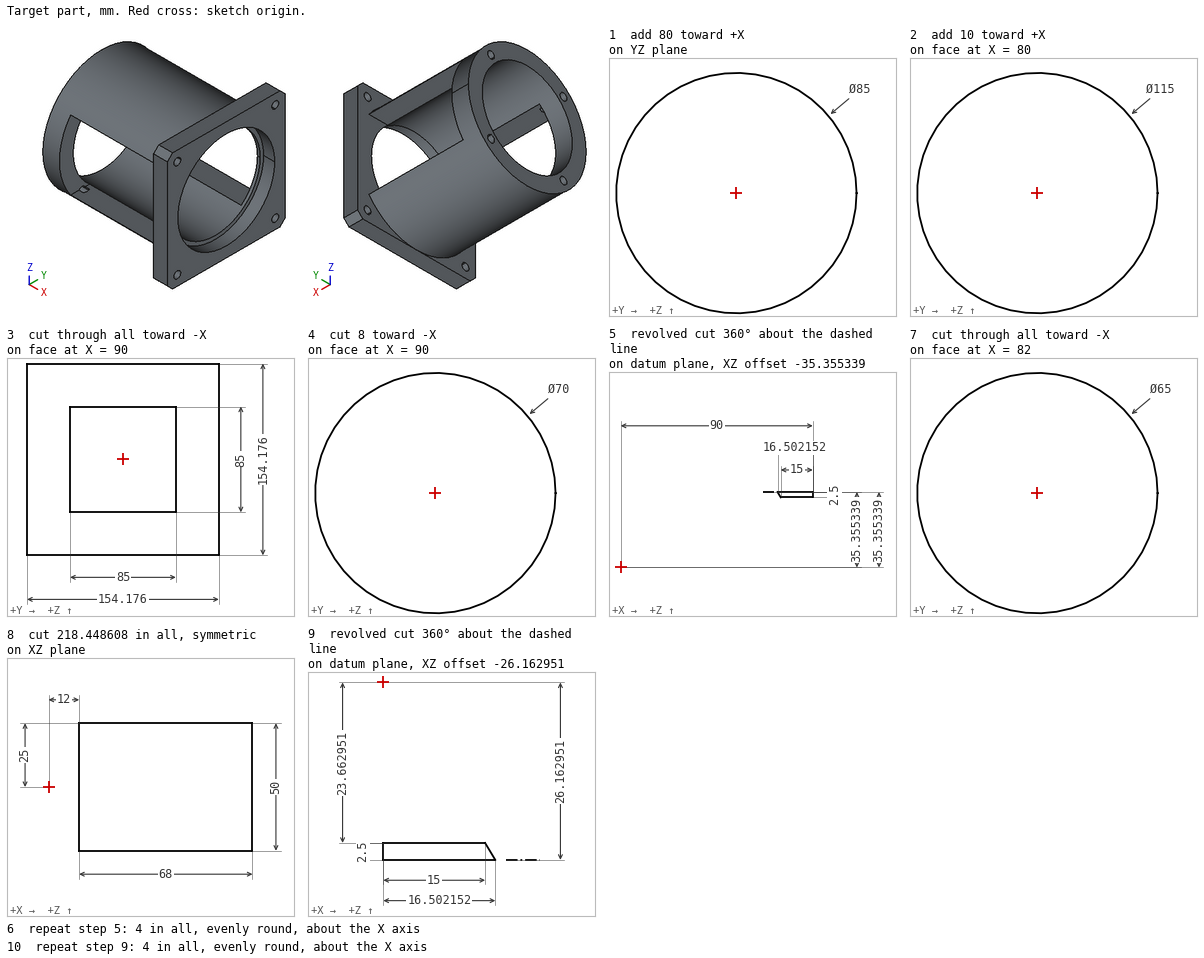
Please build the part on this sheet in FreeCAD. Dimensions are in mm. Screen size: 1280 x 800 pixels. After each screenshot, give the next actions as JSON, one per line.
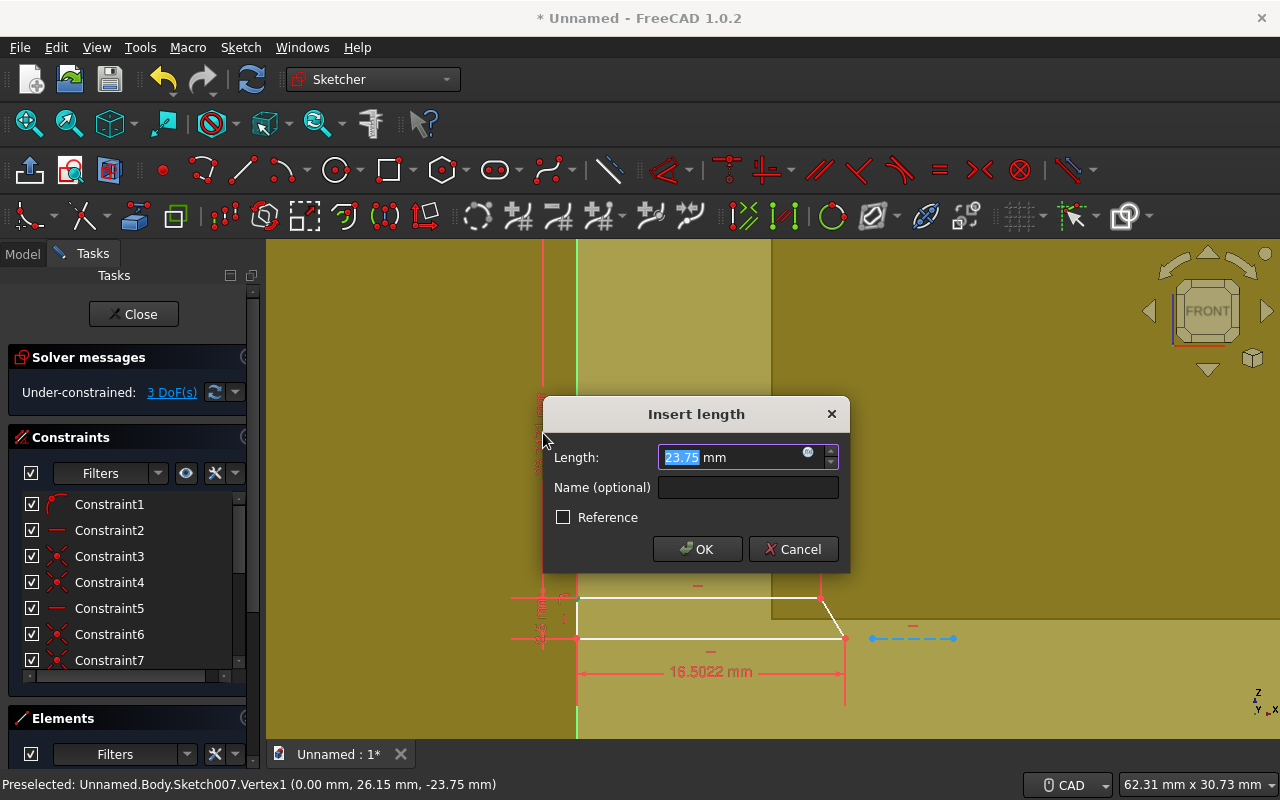
{"action": "type", "text": "23.662951"}
{"action": "key", "text": "Return"}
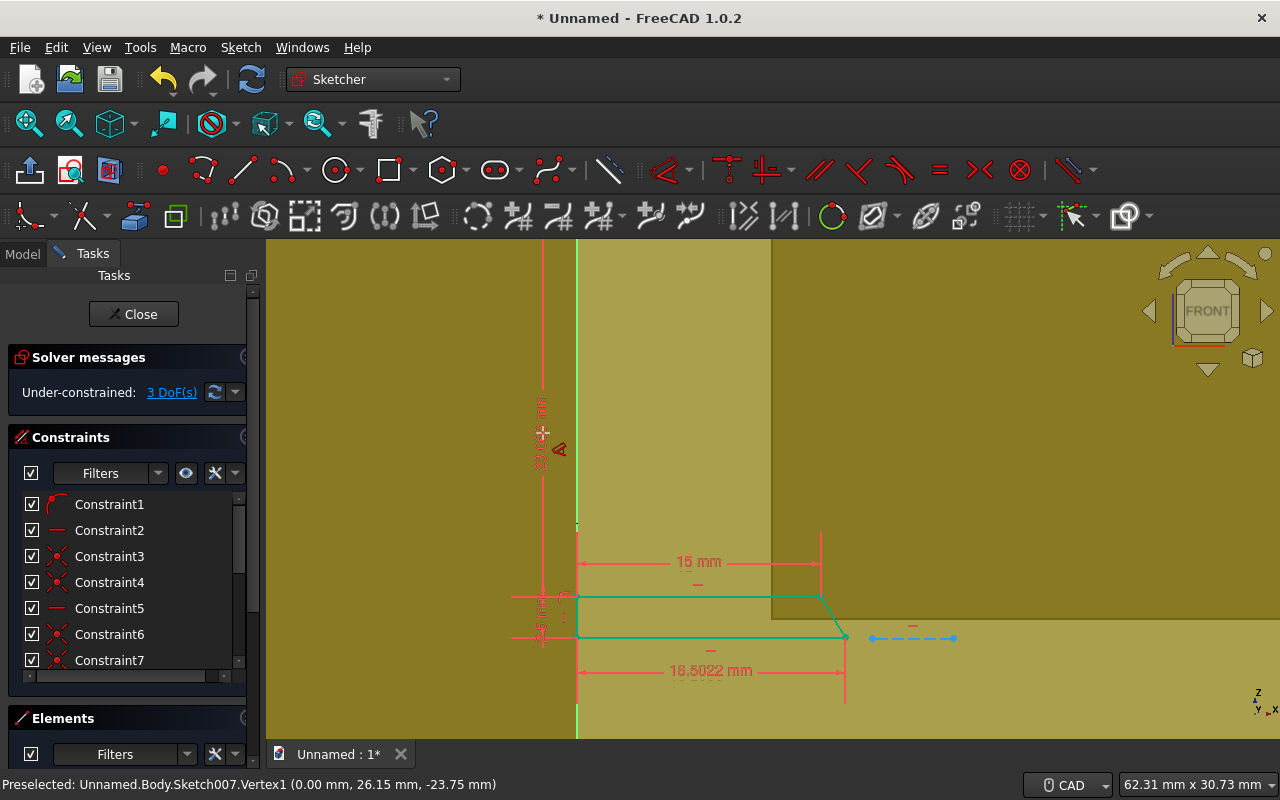
{"action": "left_click", "coordinate": [873, 638]}
{"action": "left_click", "coordinate": [543, 453]}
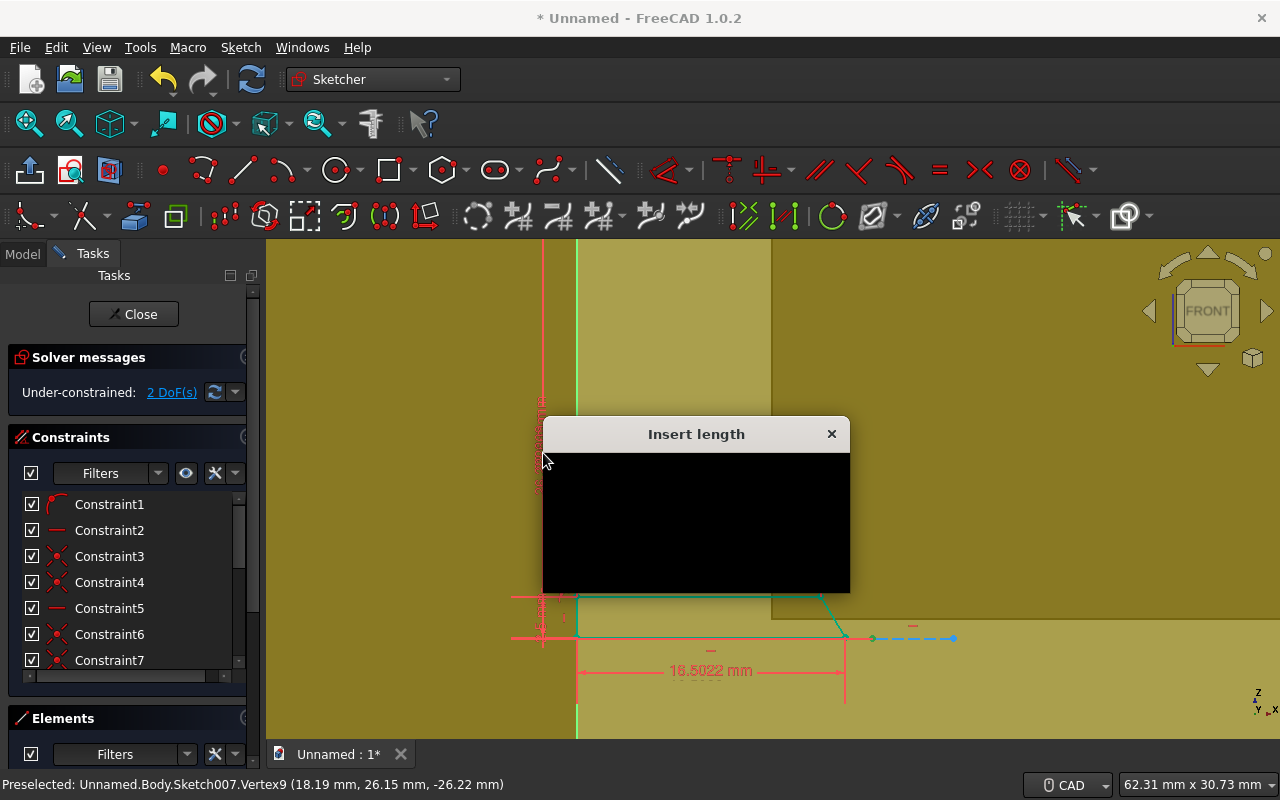
{"action": "type", "text": "26.162951"}
{"action": "key", "text": "Return"}
{"action": "key", "text": "Escape"}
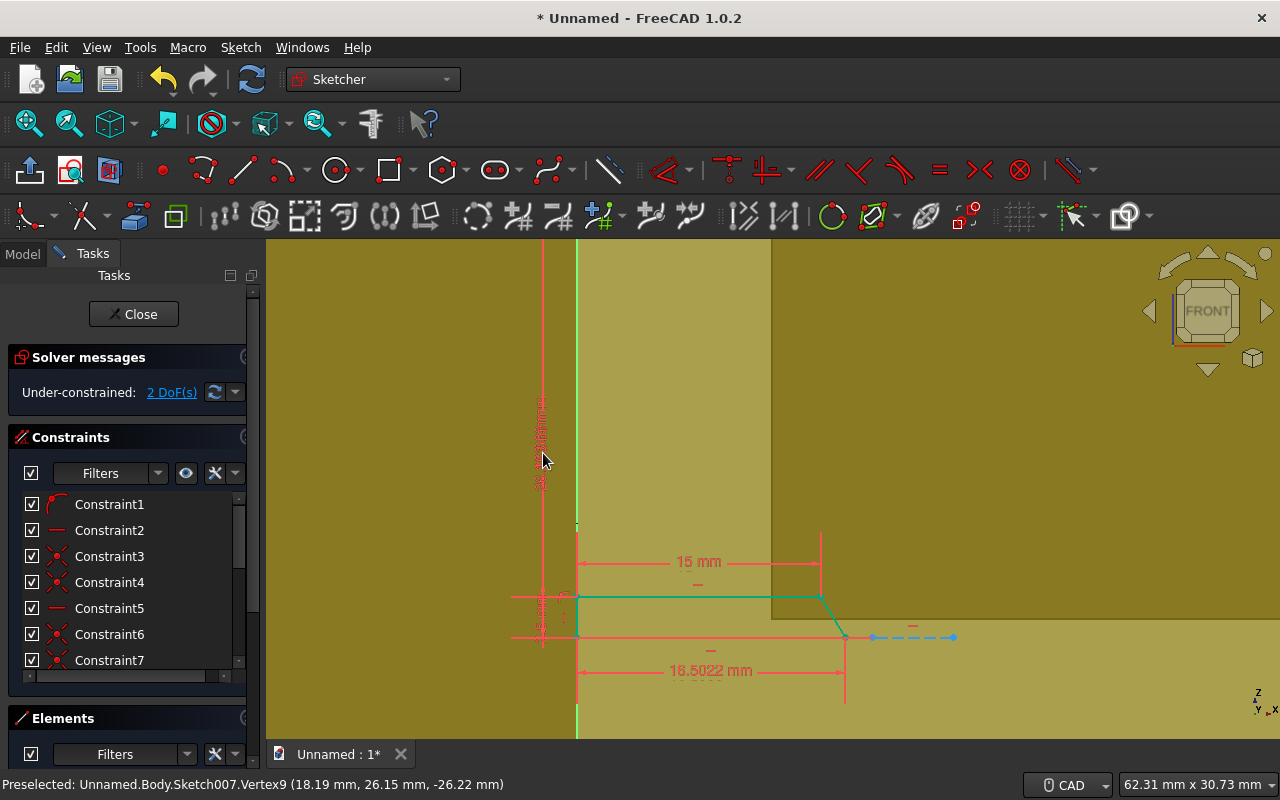
{"action": "left_click", "coordinate": [134, 314]}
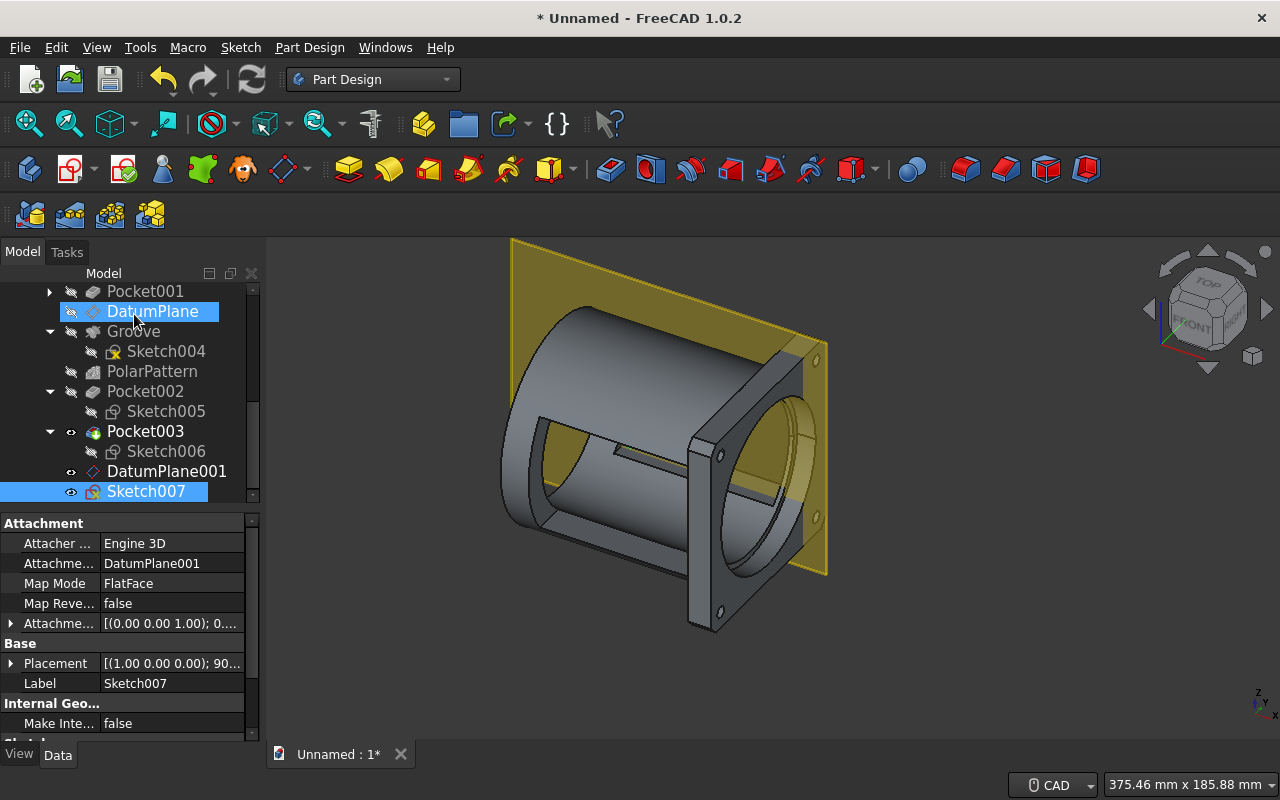
{"action": "left_click", "coordinate": [692, 170]}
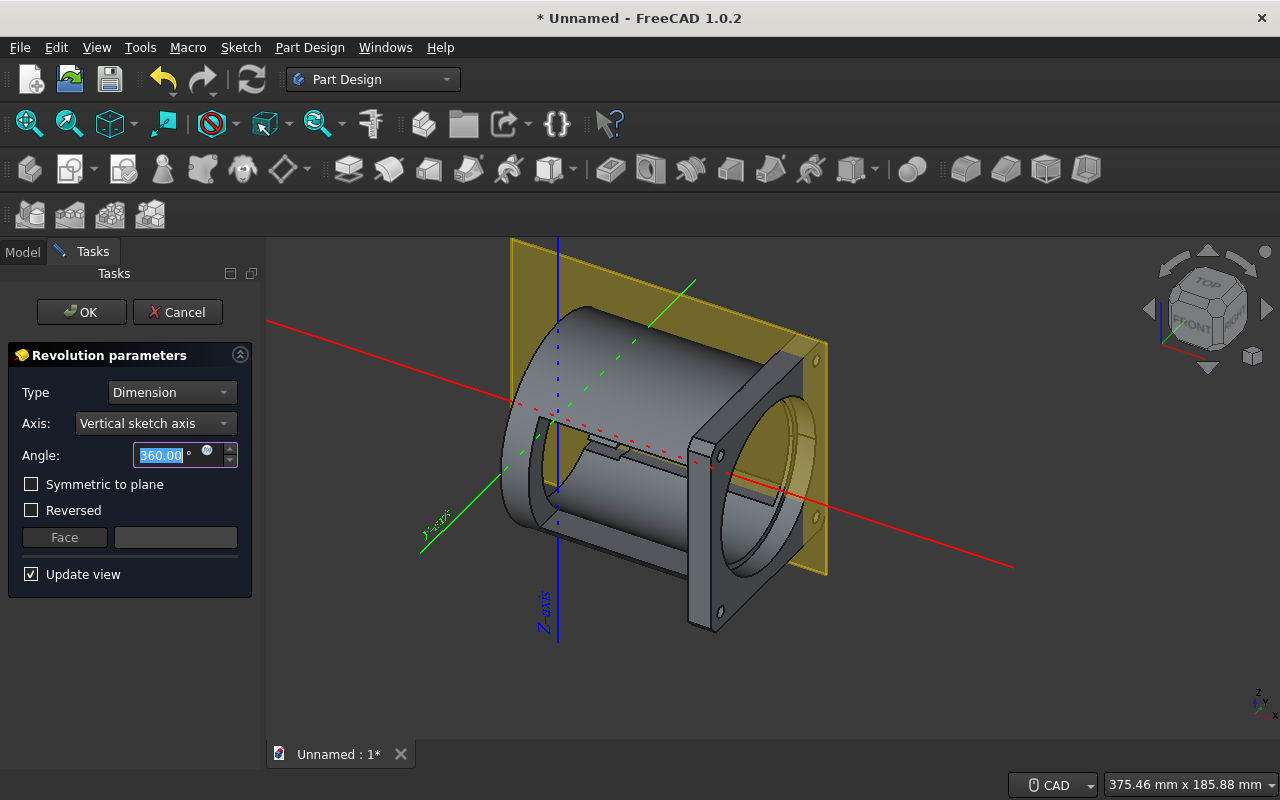
{"action": "left_click", "coordinate": [156, 424]}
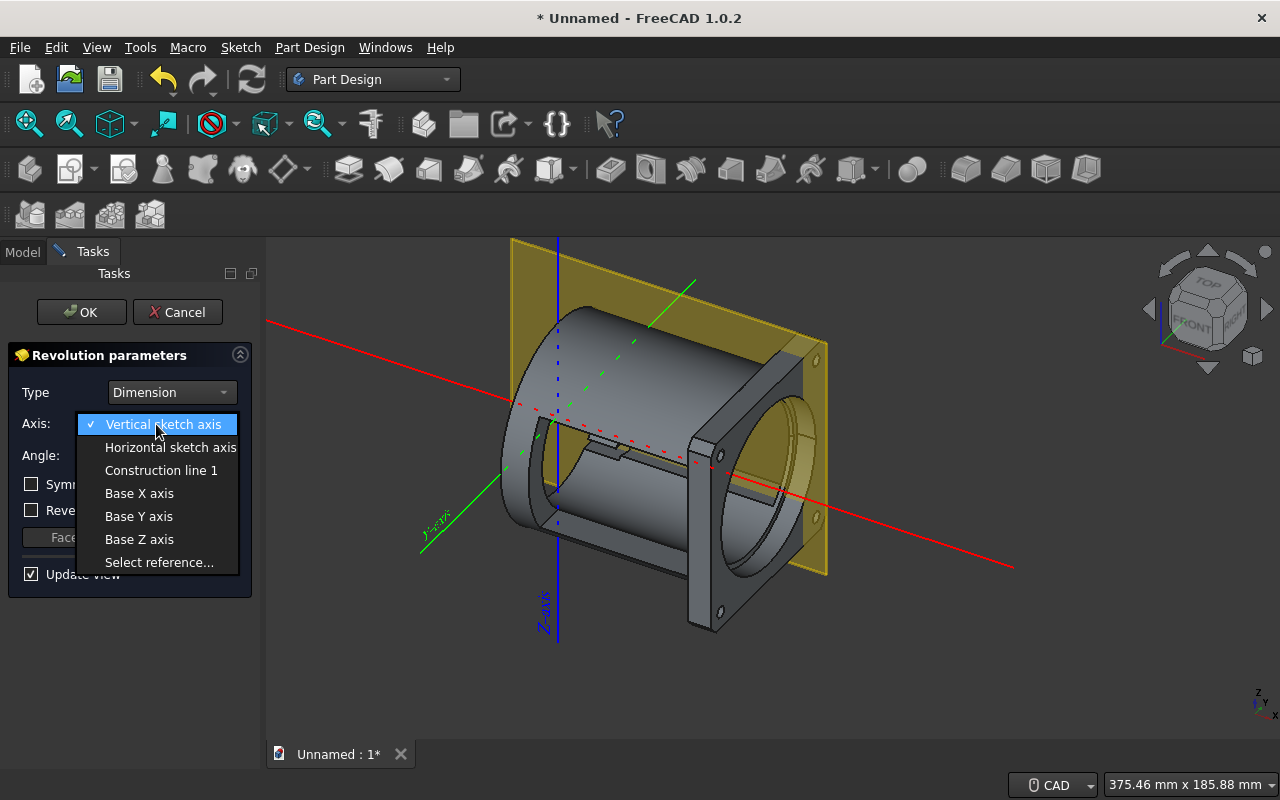
{"action": "left_click", "coordinate": [156, 470]}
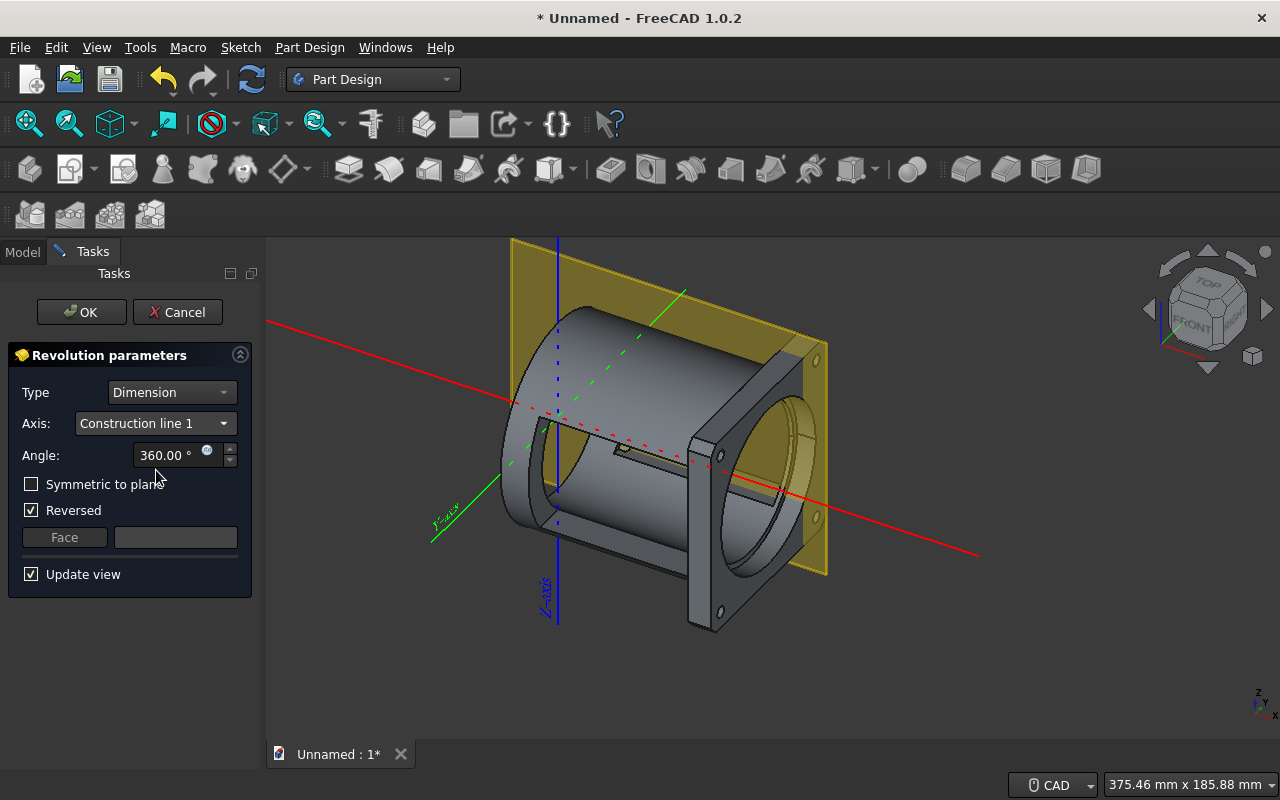
{"action": "left_click", "coordinate": [82, 312]}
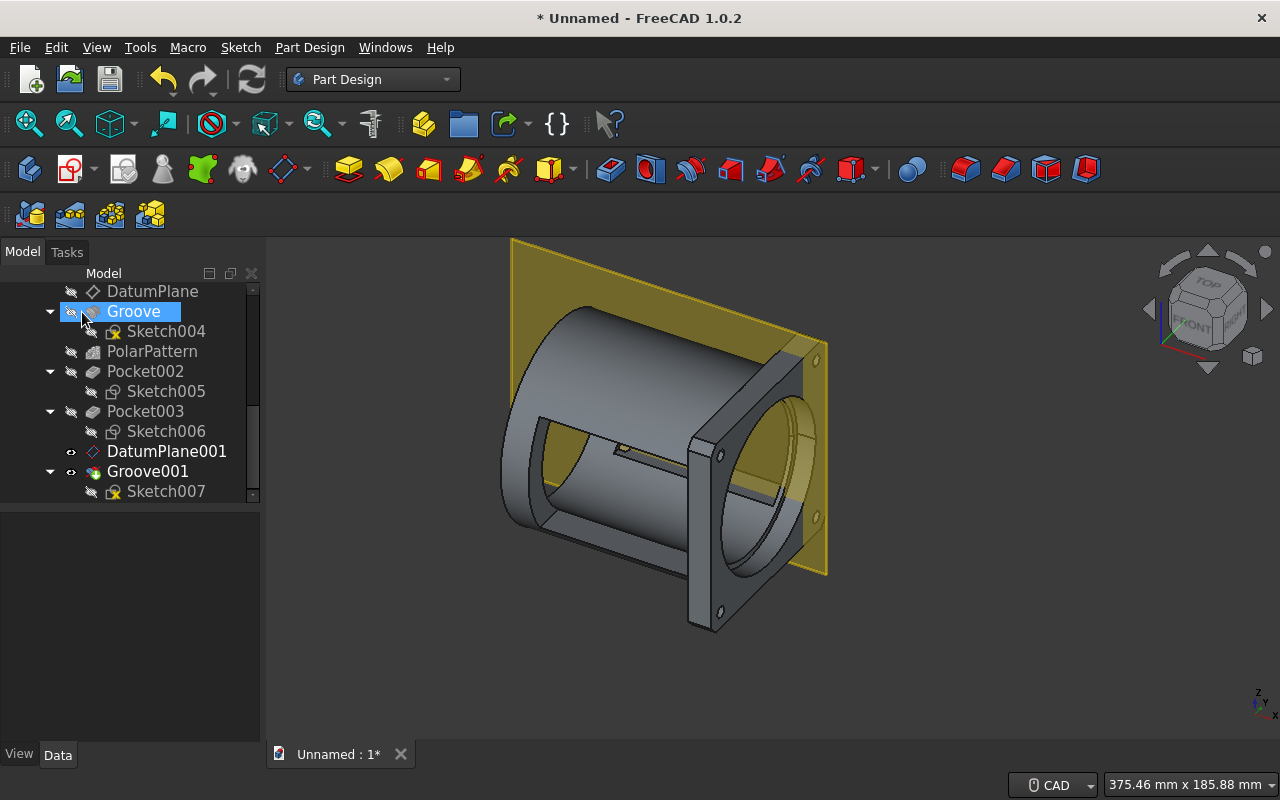
{"action": "left_click", "coordinate": [116, 452]}
{"action": "key", "text": "space"}